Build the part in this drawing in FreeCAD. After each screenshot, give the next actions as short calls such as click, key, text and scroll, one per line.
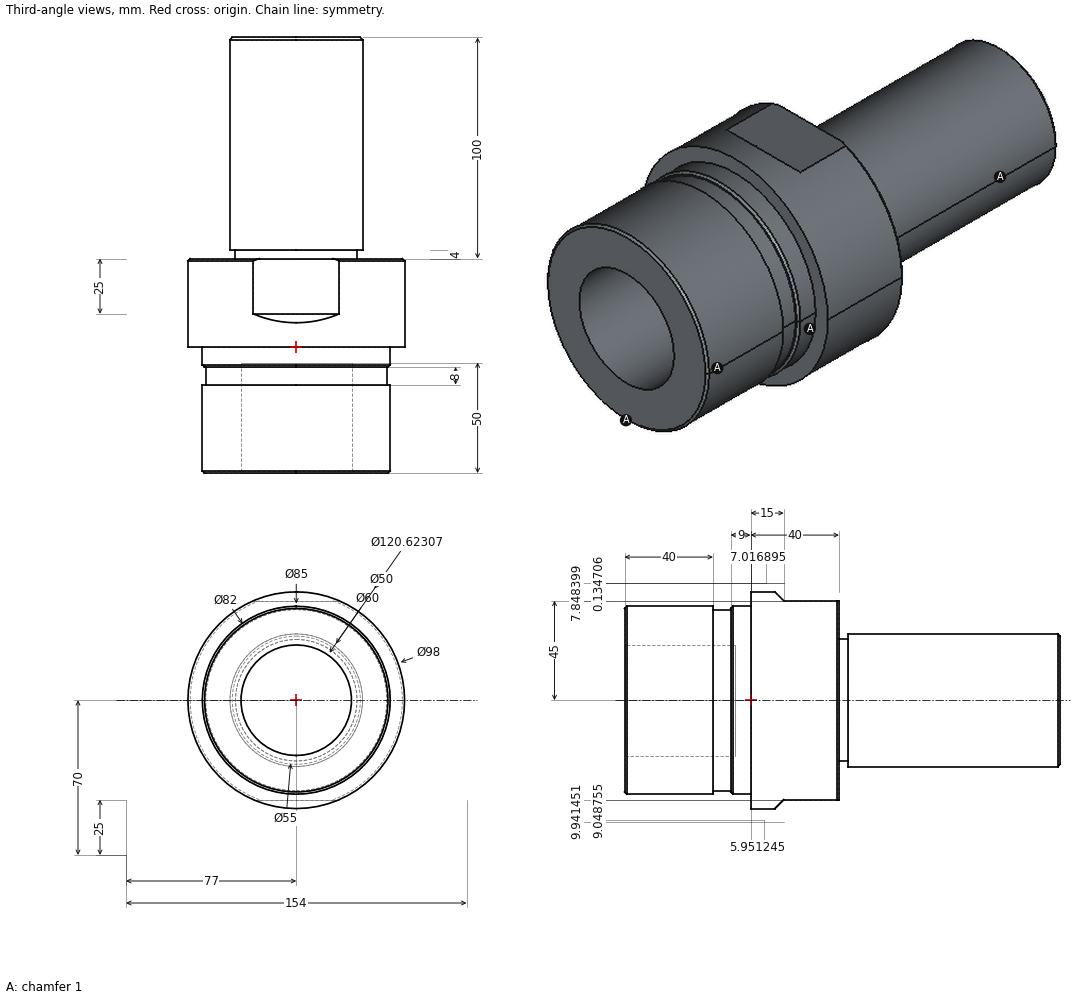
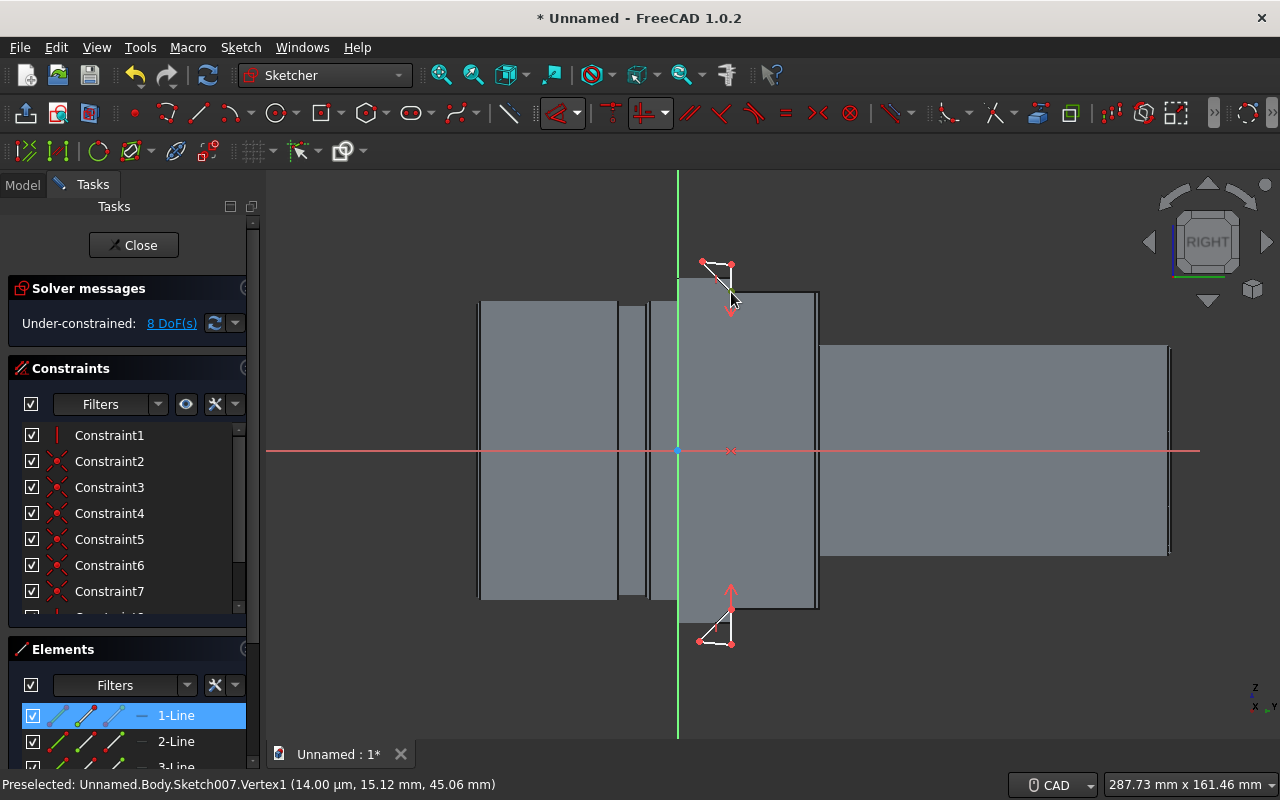
key(l)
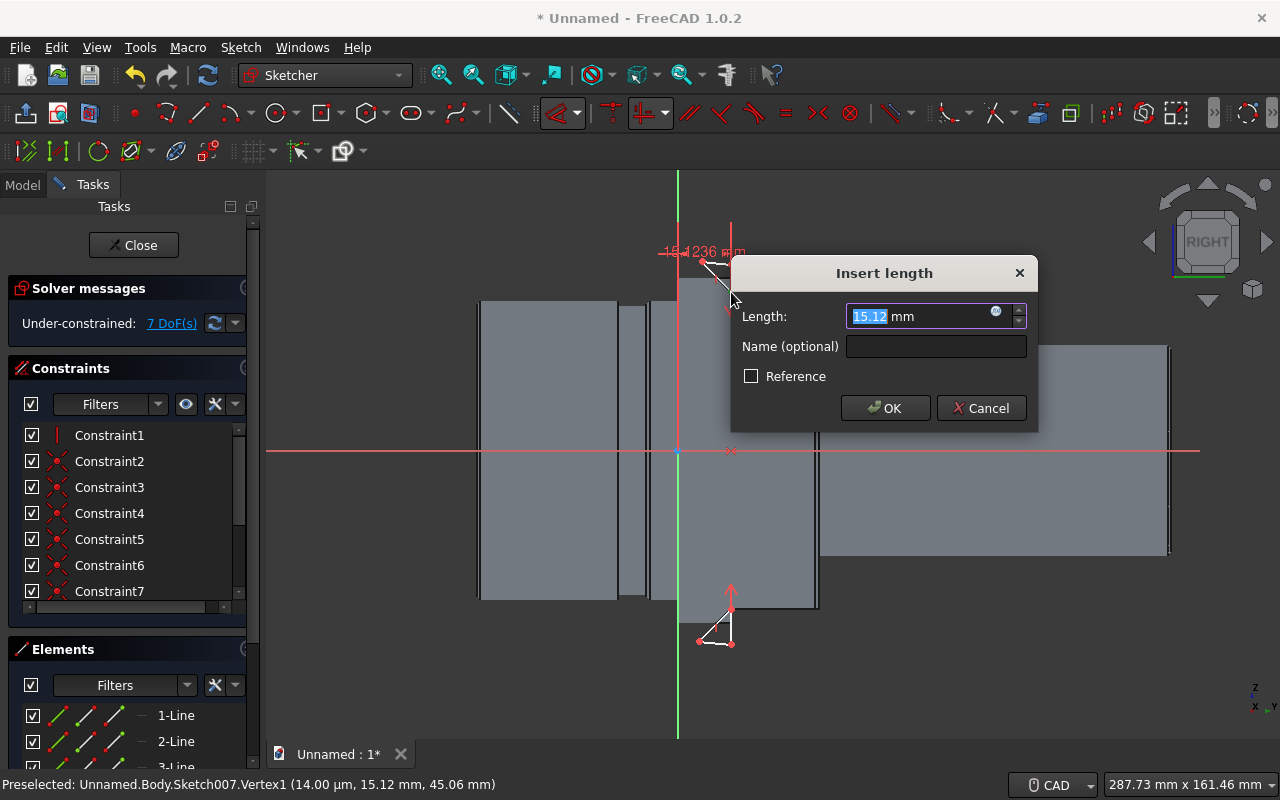
text(15)
key(Return)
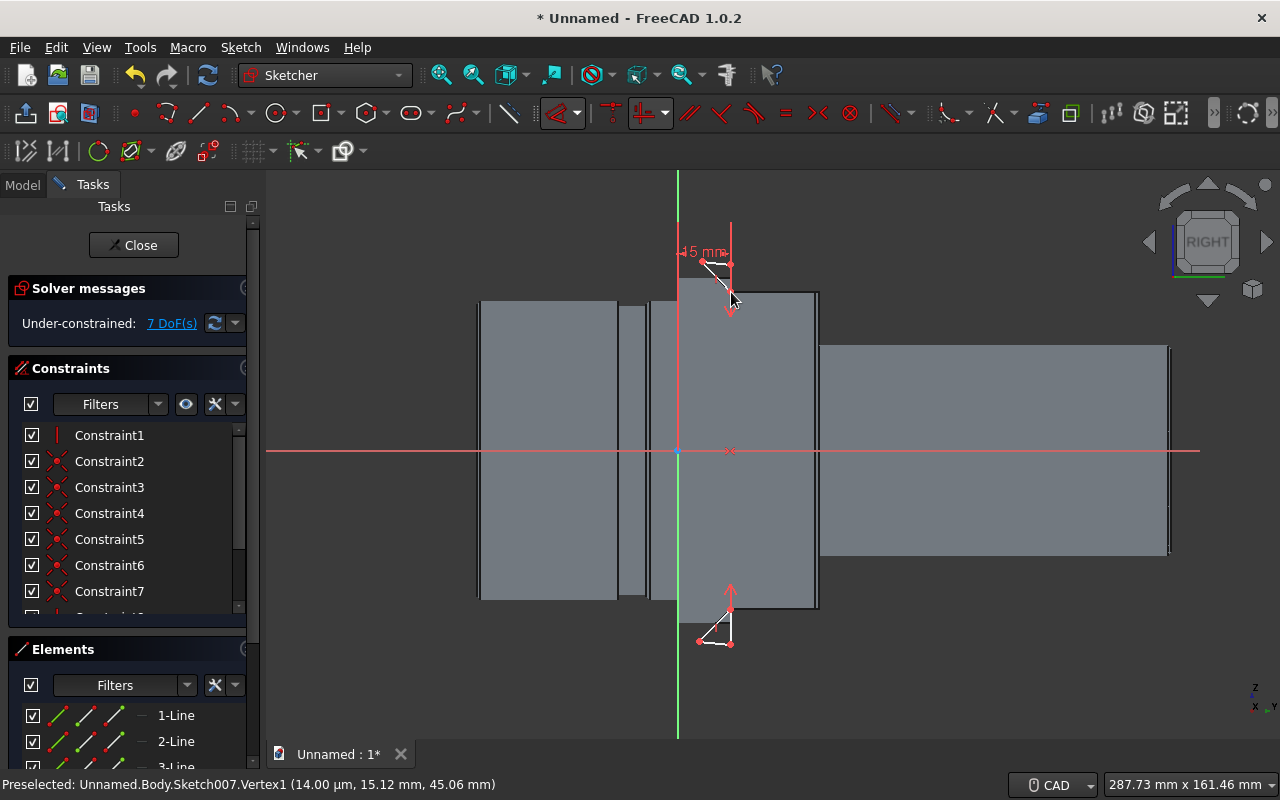
click(731, 292)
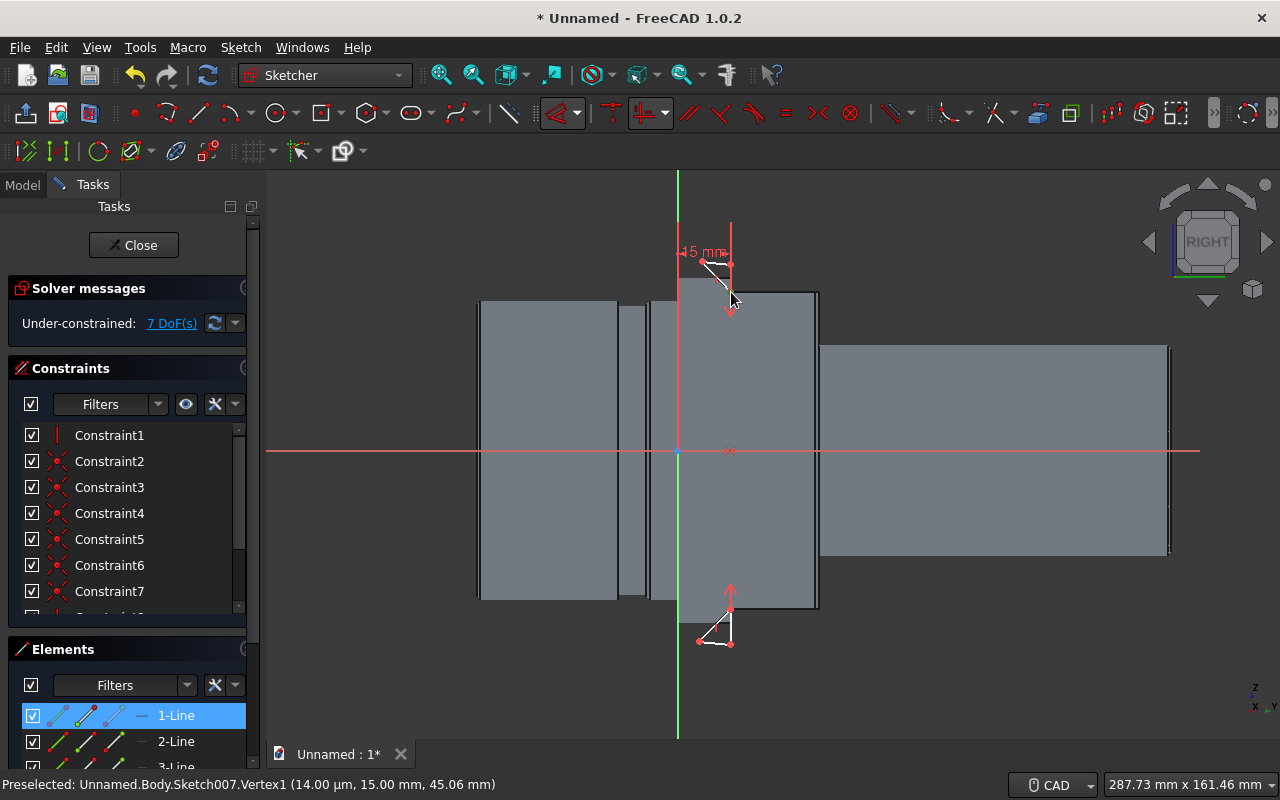
key(i)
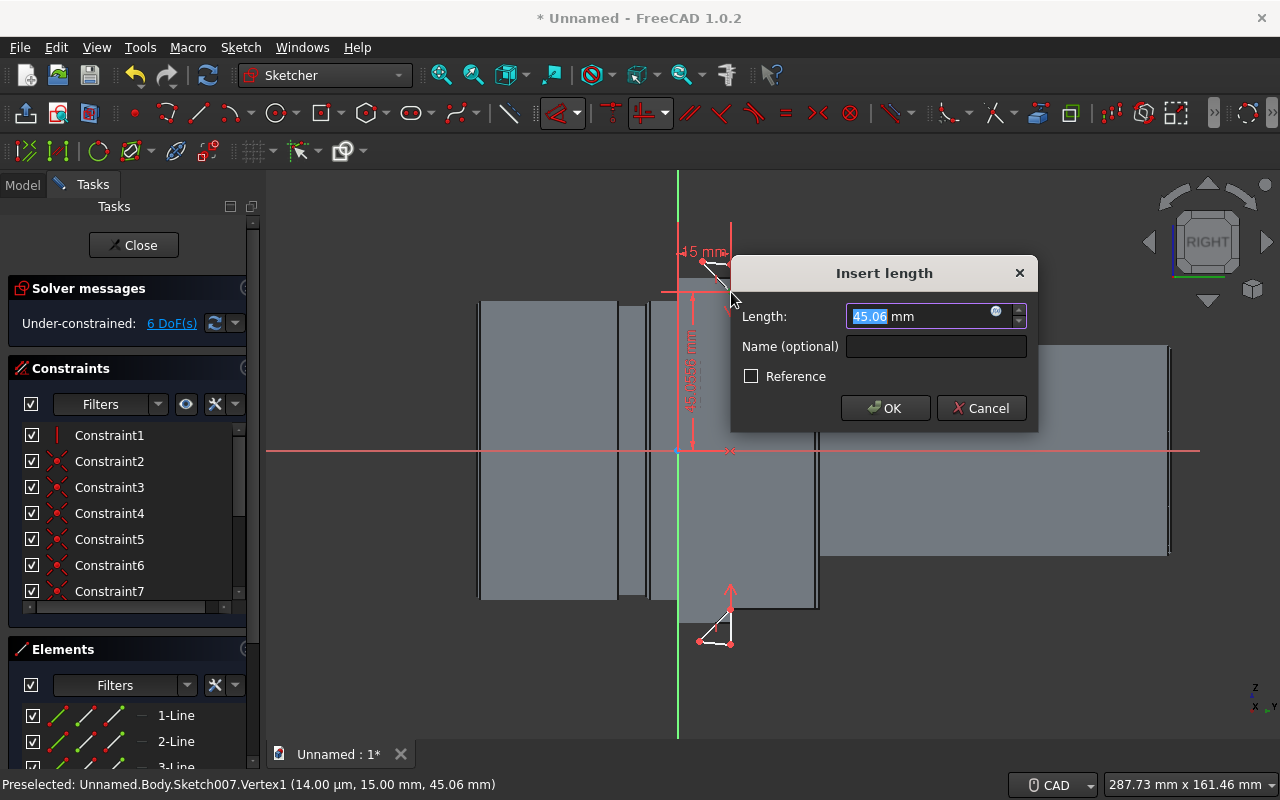
text(45)
key(Return)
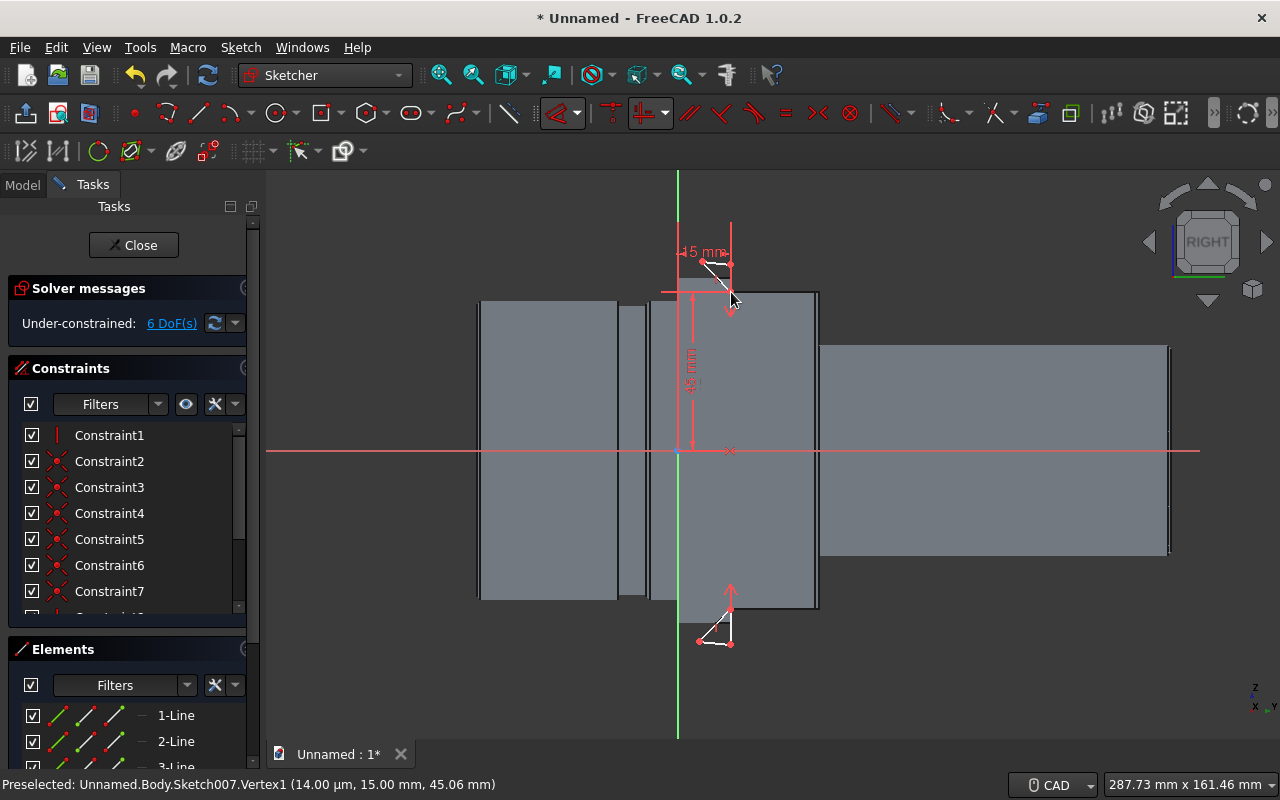
scroll(731, 276, up, 2)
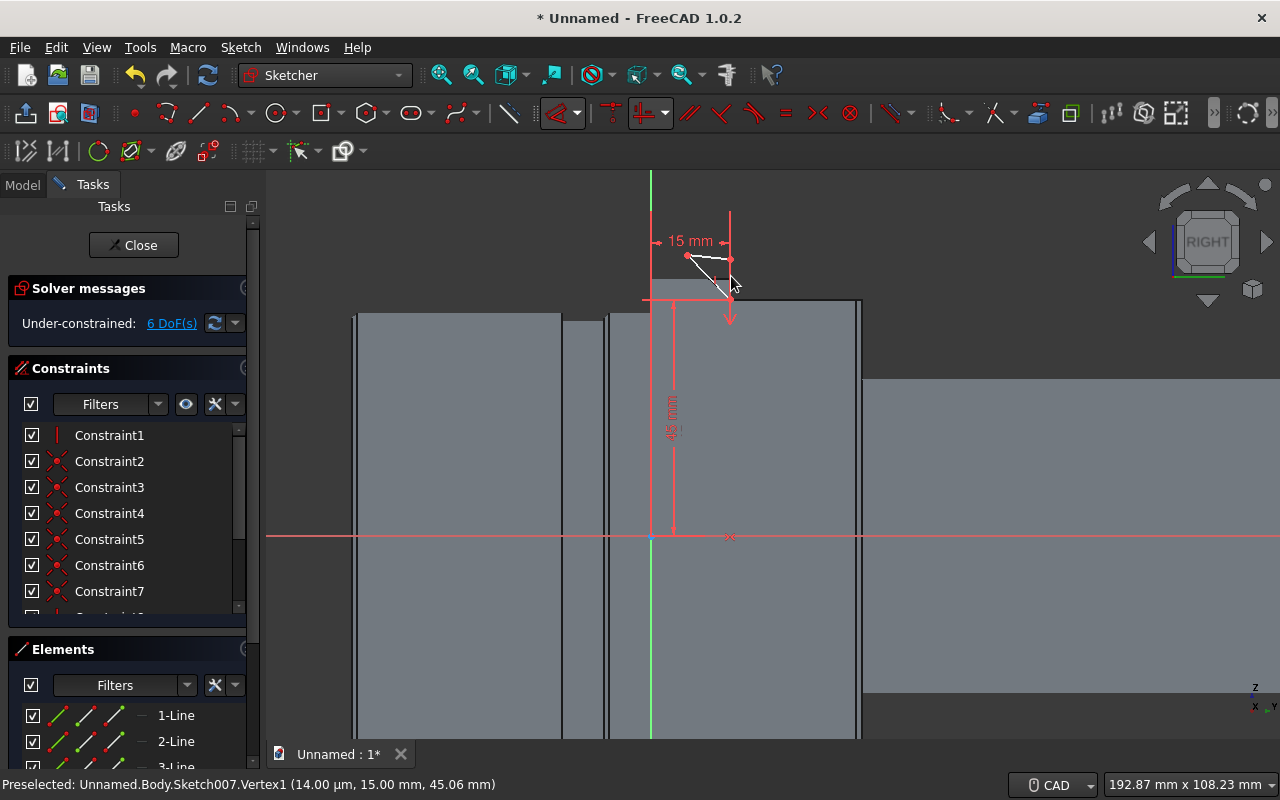
click(730, 276)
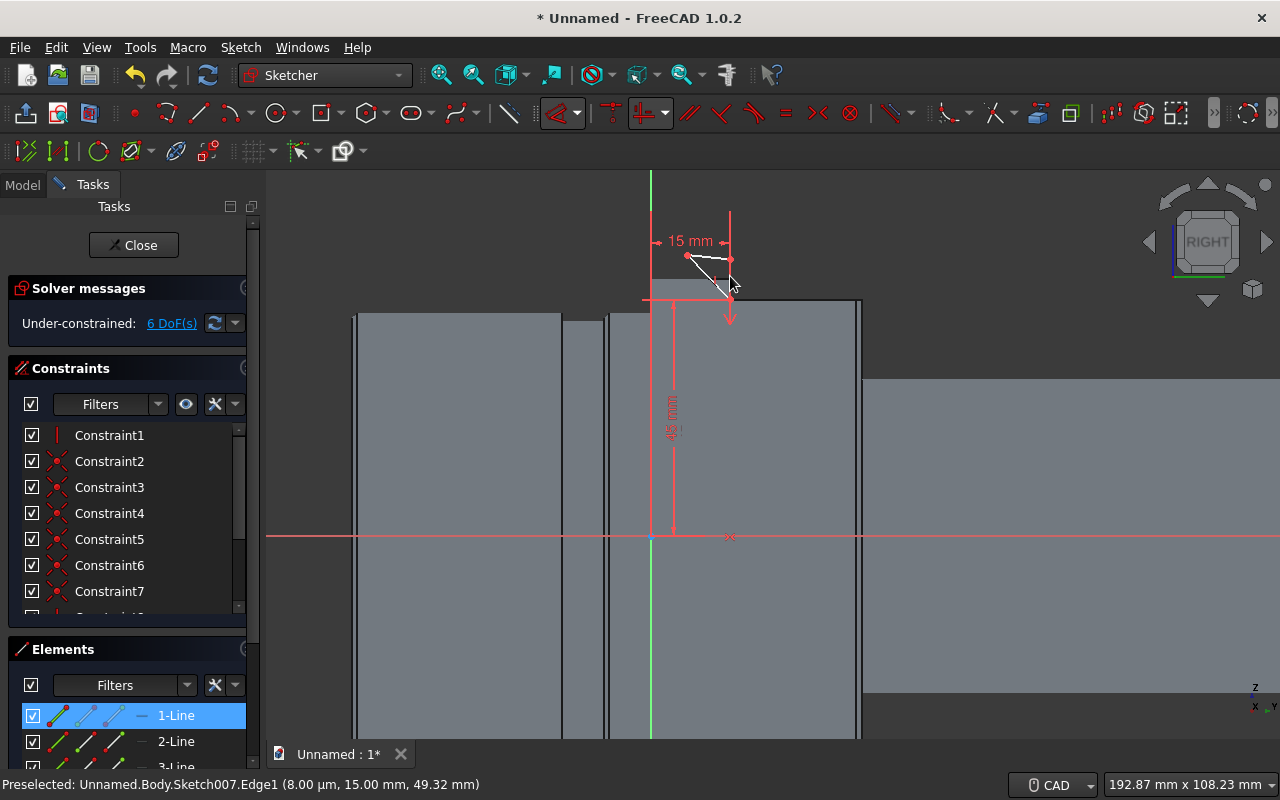
click(580, 114)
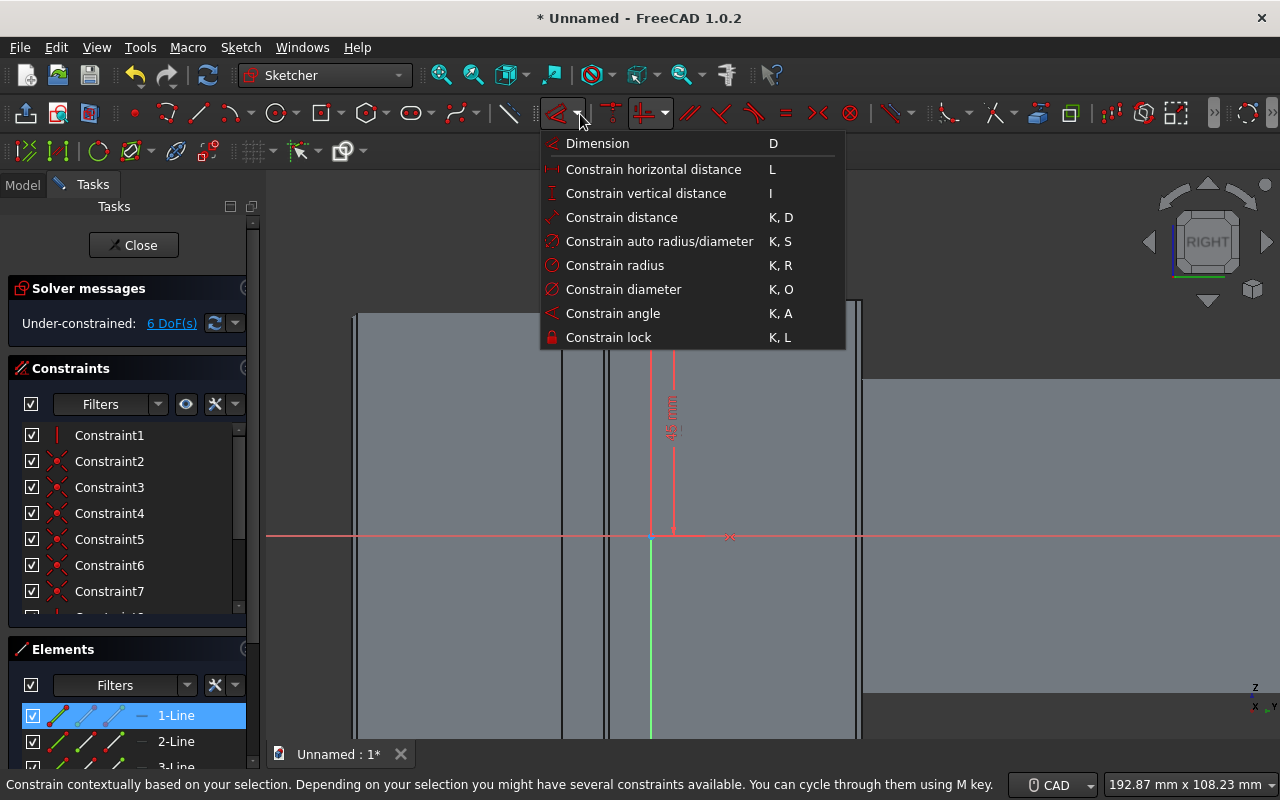
click(693, 193)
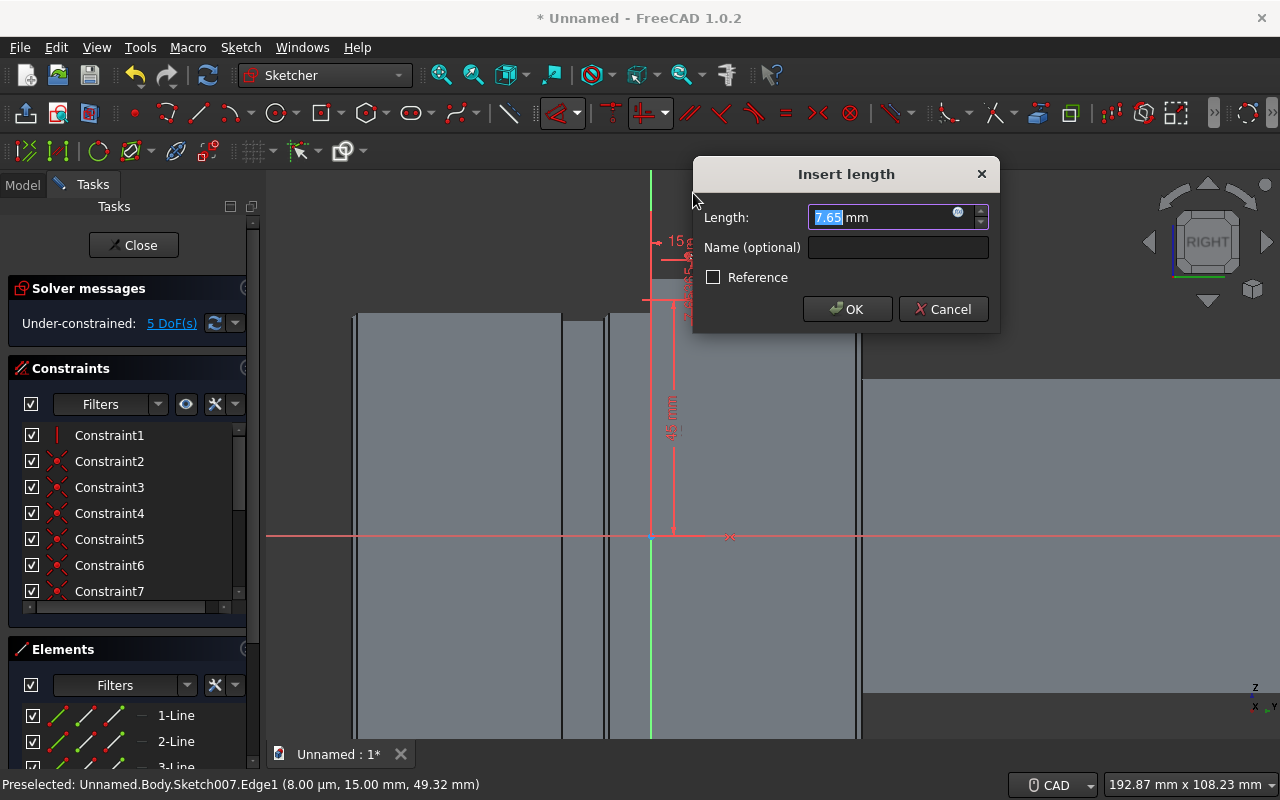
text(7.848399)
key(Return)